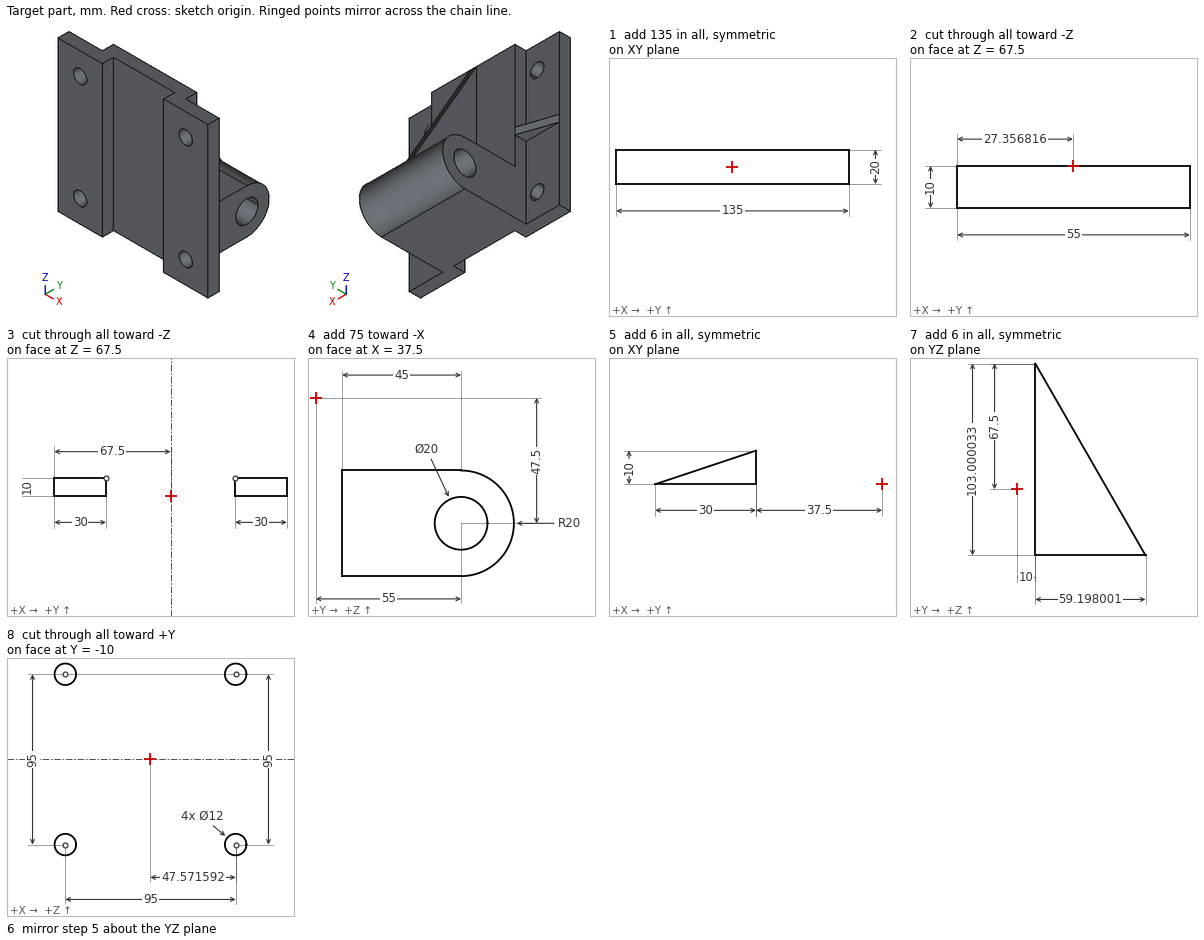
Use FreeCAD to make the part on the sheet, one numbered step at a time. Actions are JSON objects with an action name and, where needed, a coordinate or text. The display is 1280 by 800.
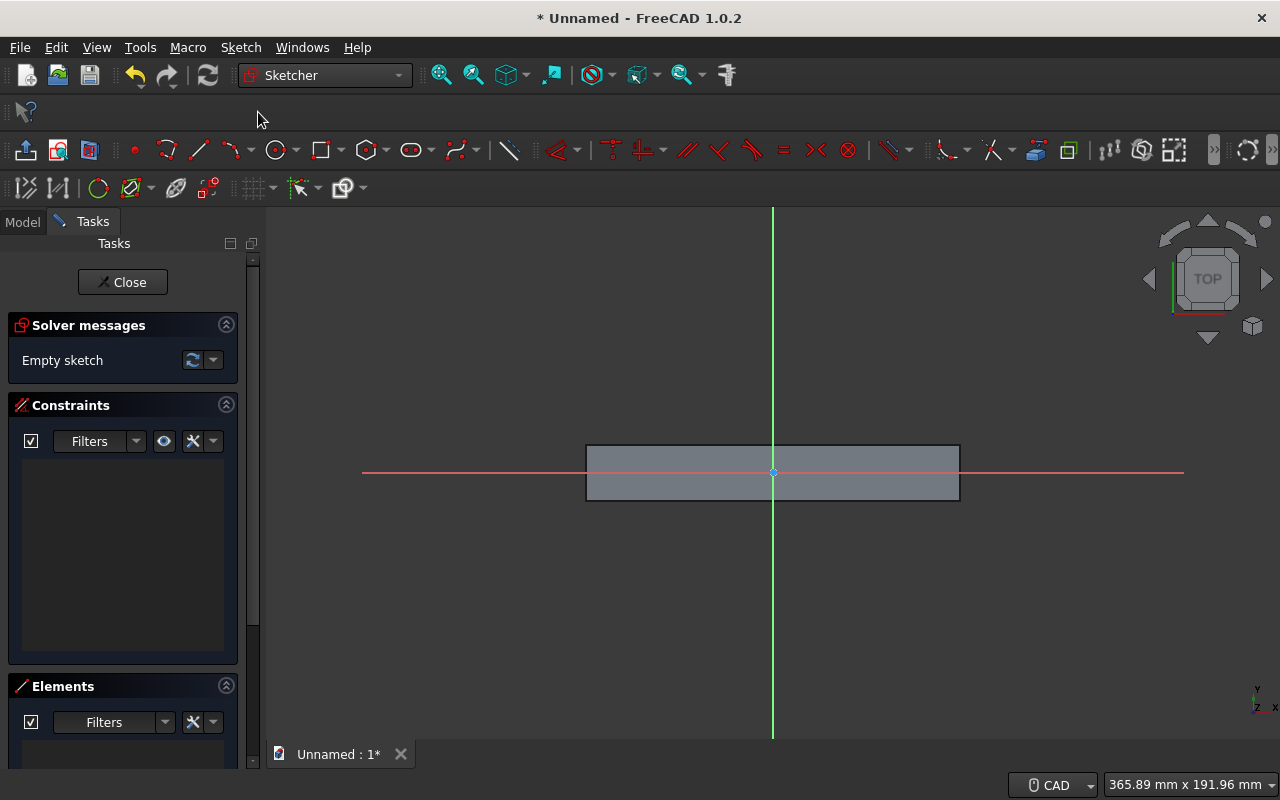
{"action": "scroll", "coordinate": [796, 491], "scroll_direction": "up", "scroll_amount": 7}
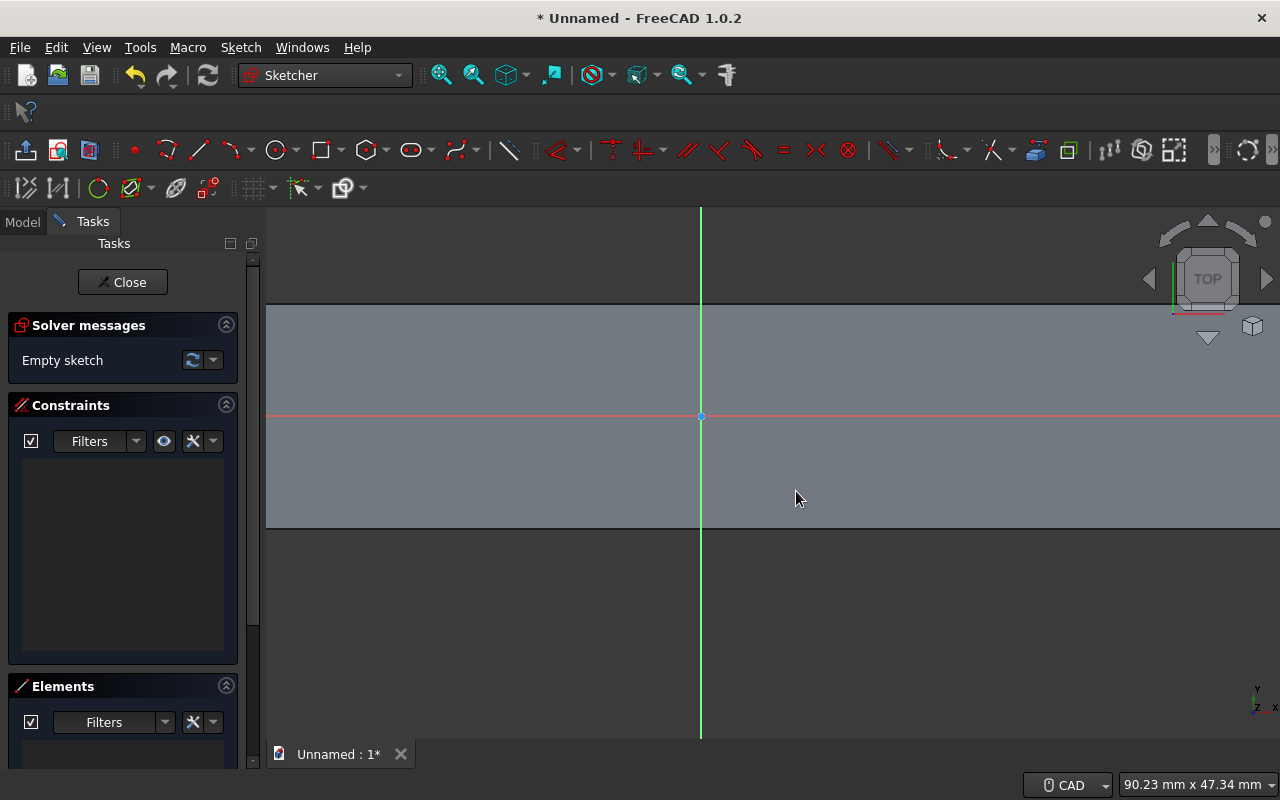
{"action": "left_click", "coordinate": [322, 150]}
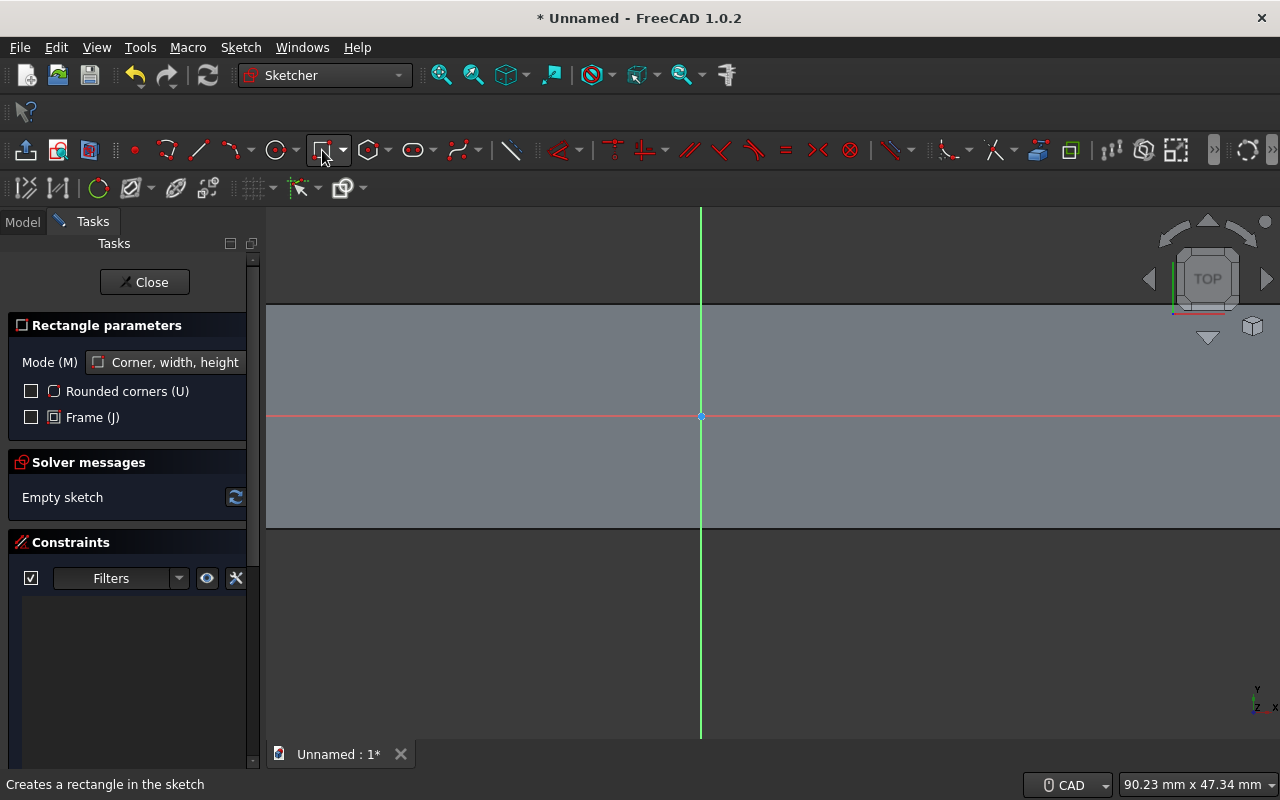
{"action": "left_click", "coordinate": [394, 416]}
{"action": "left_click", "coordinate": [1012, 529]}
{"action": "key", "text": "Escape"}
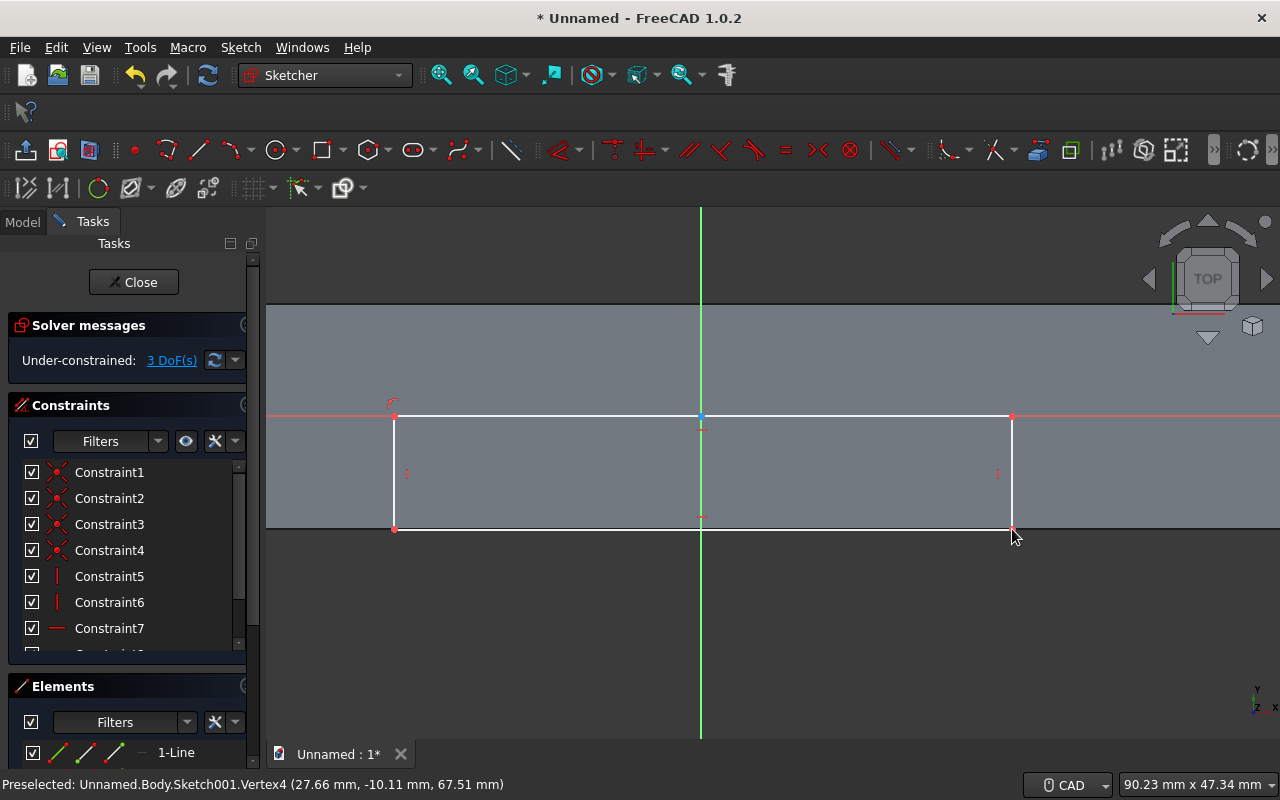
{"action": "left_click", "coordinate": [558, 150]}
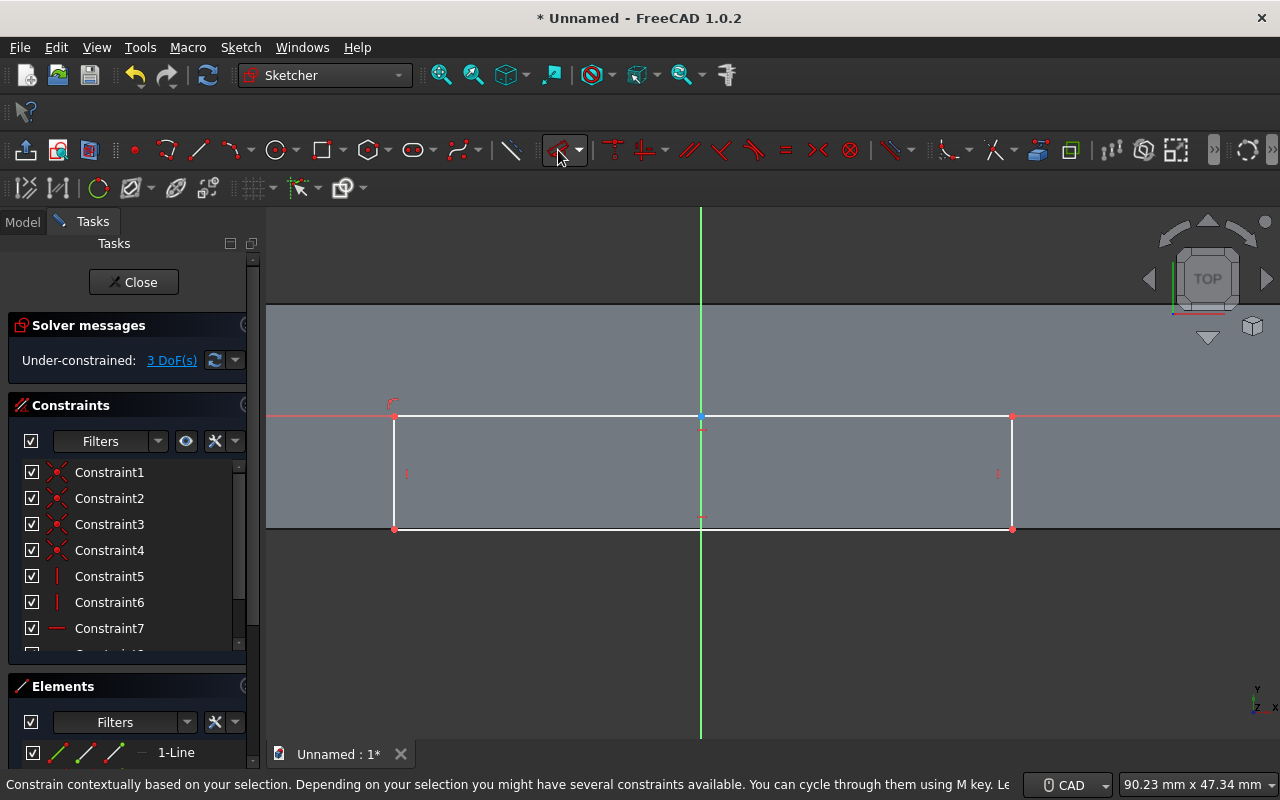
{"action": "left_click", "coordinate": [394, 450]}
{"action": "left_click", "coordinate": [360, 473]}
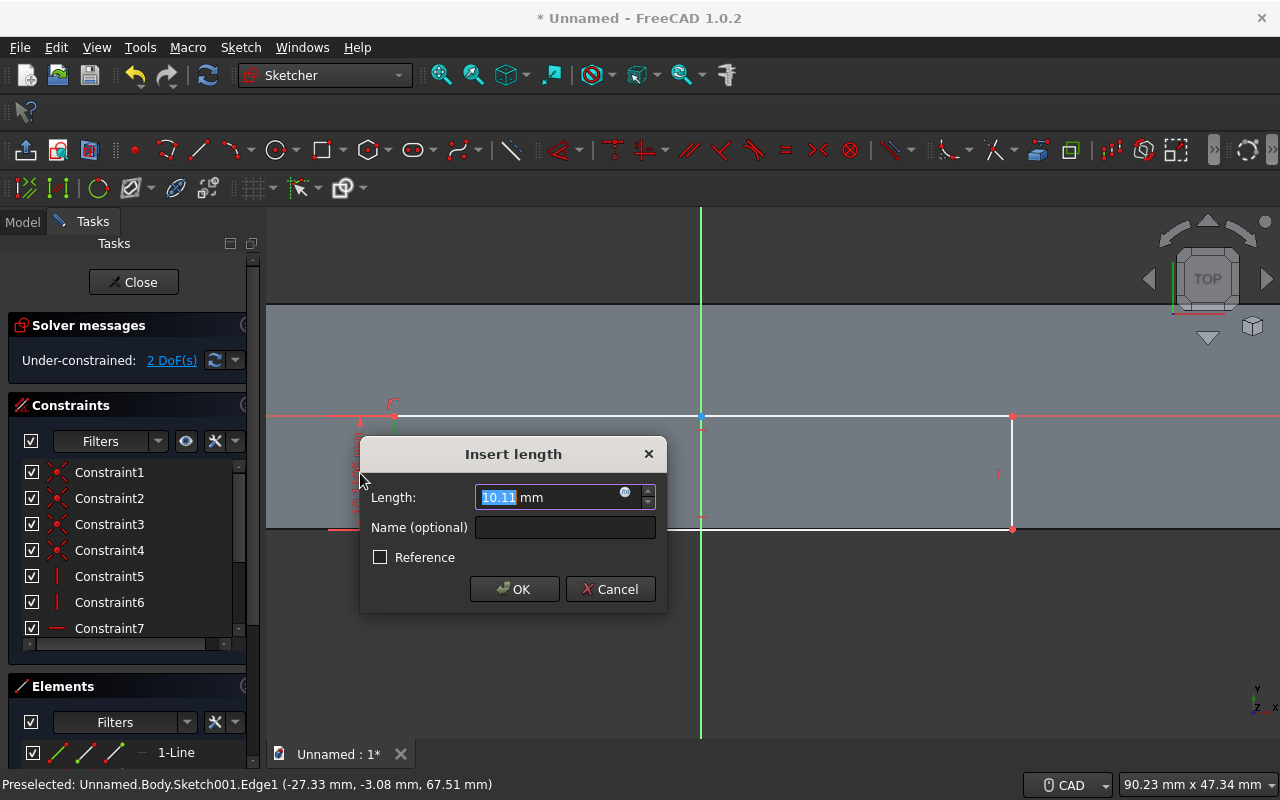
{"action": "type", "text": "10"}
{"action": "key", "text": "Return"}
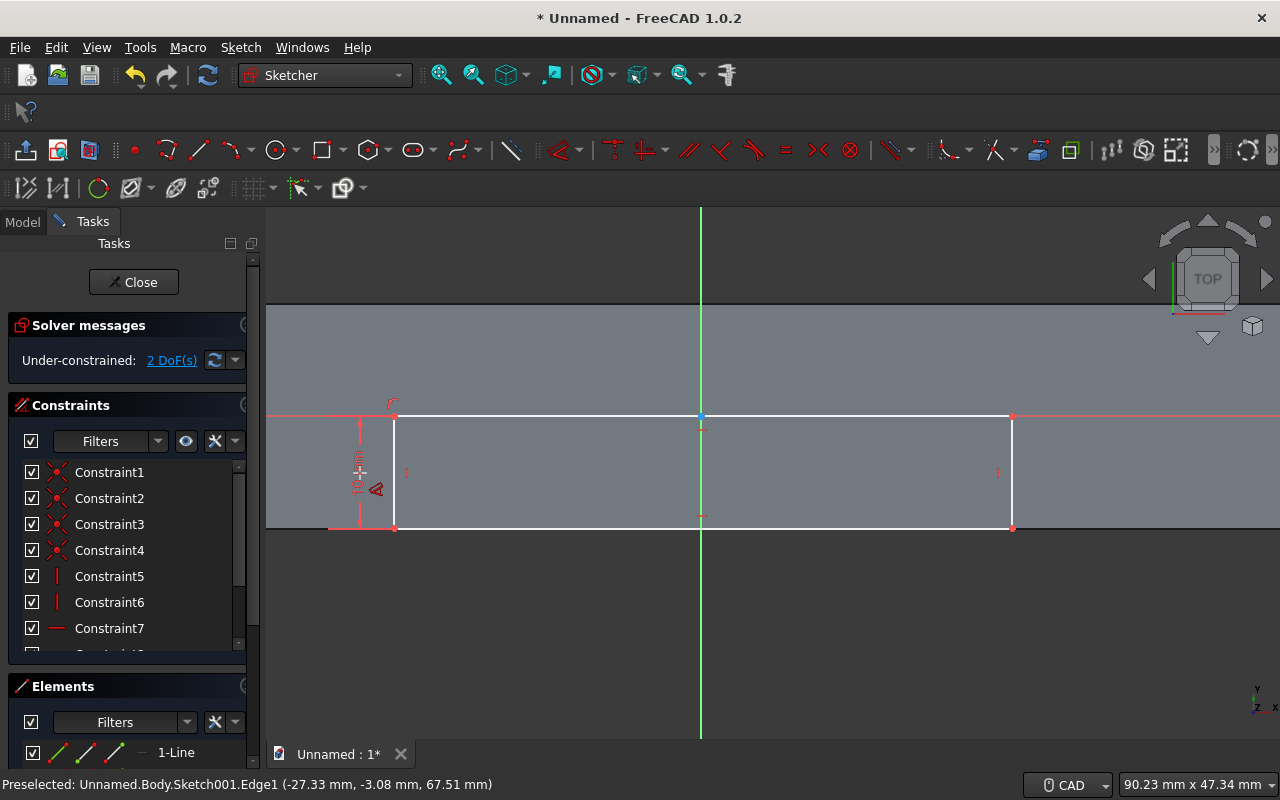
{"action": "left_click", "coordinate": [579, 529]}
{"action": "left_click", "coordinate": [561, 563]}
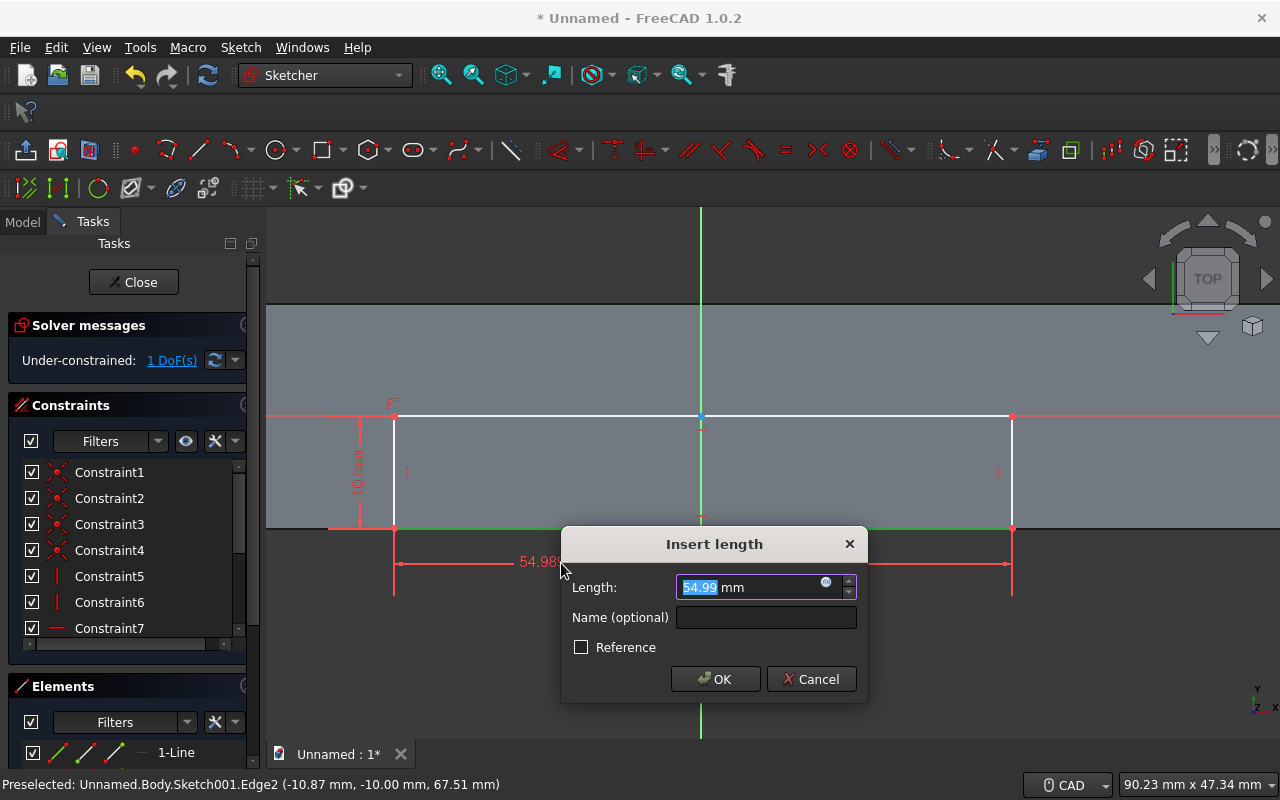
{"action": "type", "text": "55"}
{"action": "key", "text": "Return"}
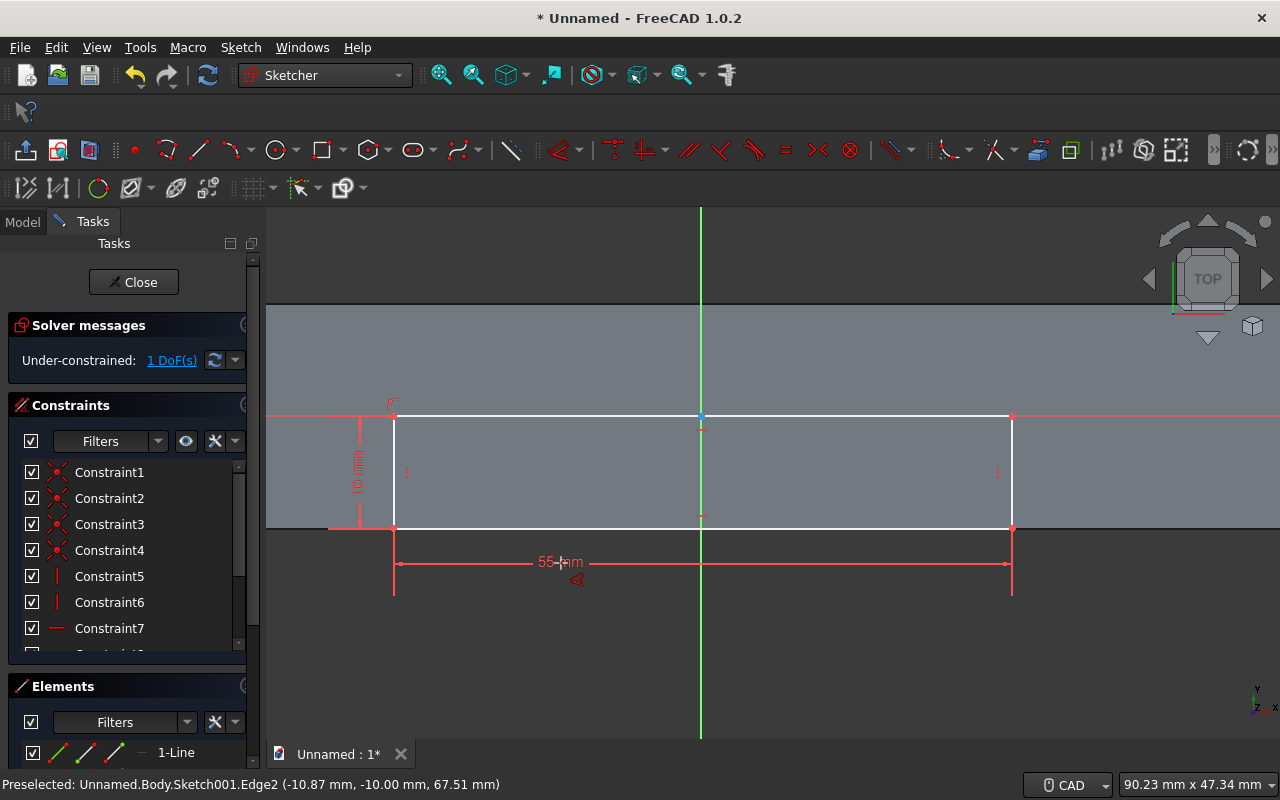
{"action": "left_click", "coordinate": [394, 416]}
{"action": "left_click", "coordinate": [548, 382]}